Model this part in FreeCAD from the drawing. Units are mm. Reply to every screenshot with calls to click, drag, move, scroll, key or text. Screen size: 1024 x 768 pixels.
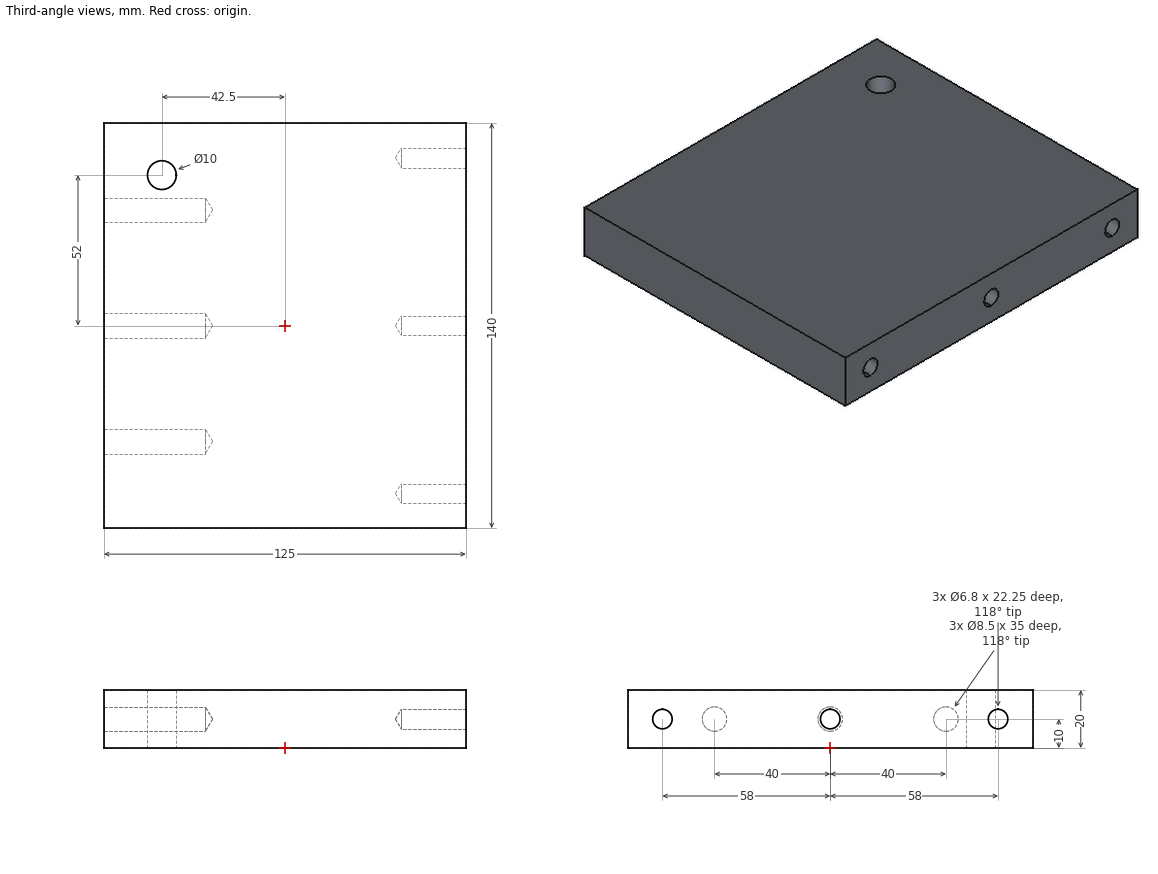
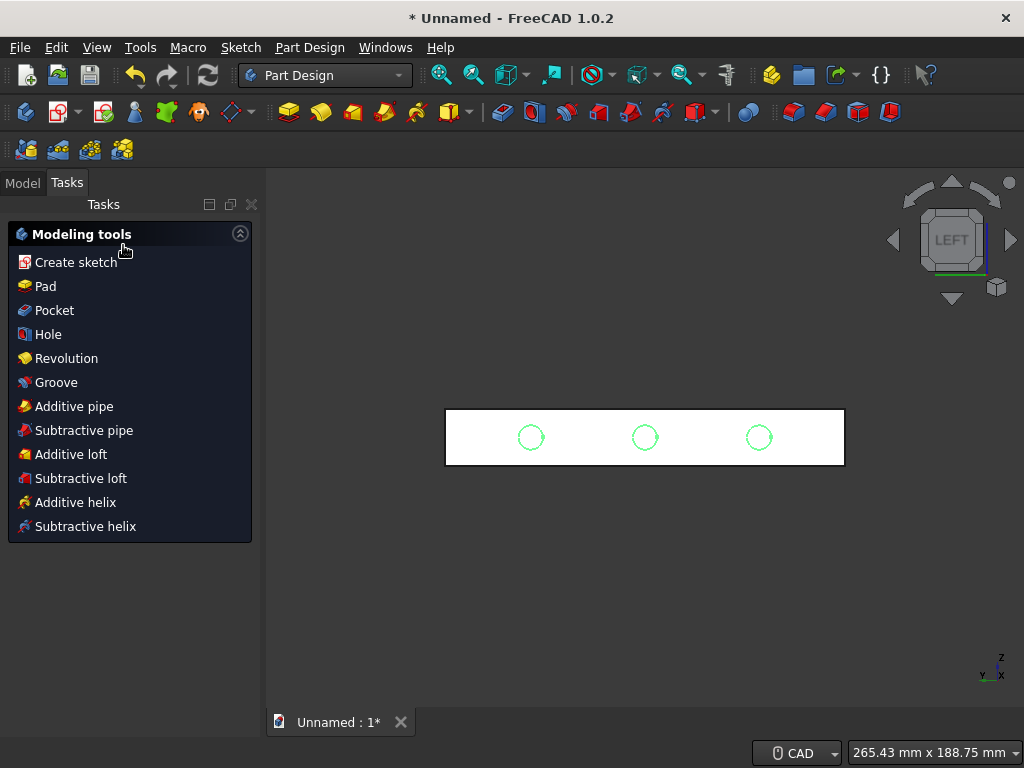
click(536, 112)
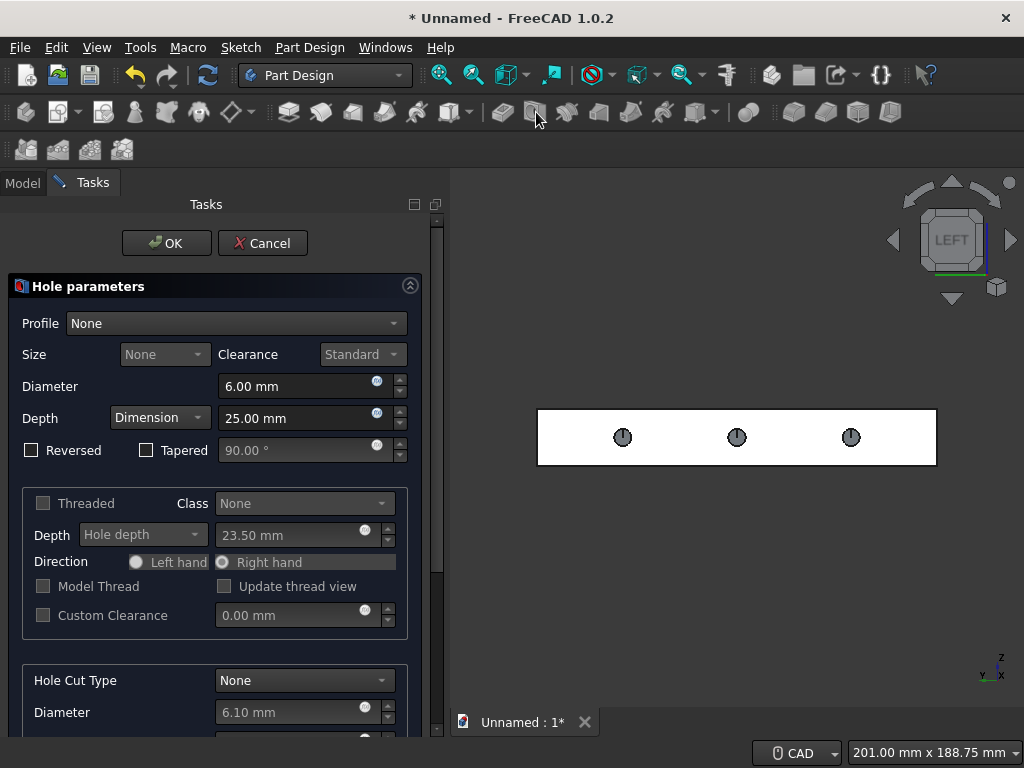
triple_click(305, 386)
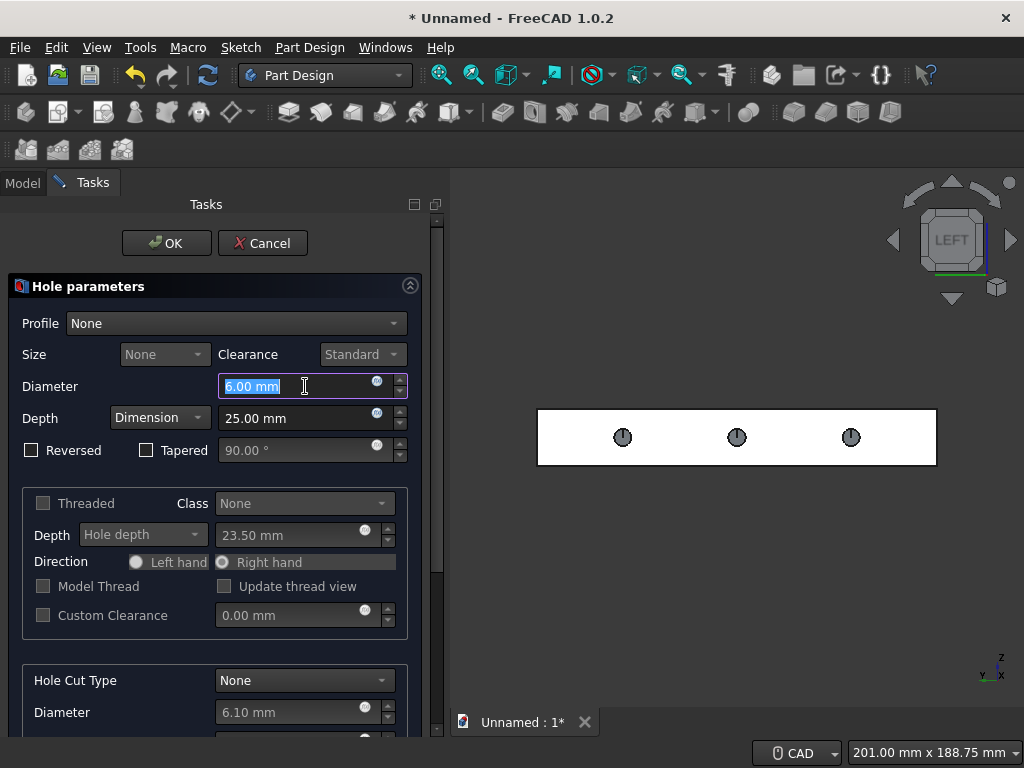
text(8.5)
key(Tab)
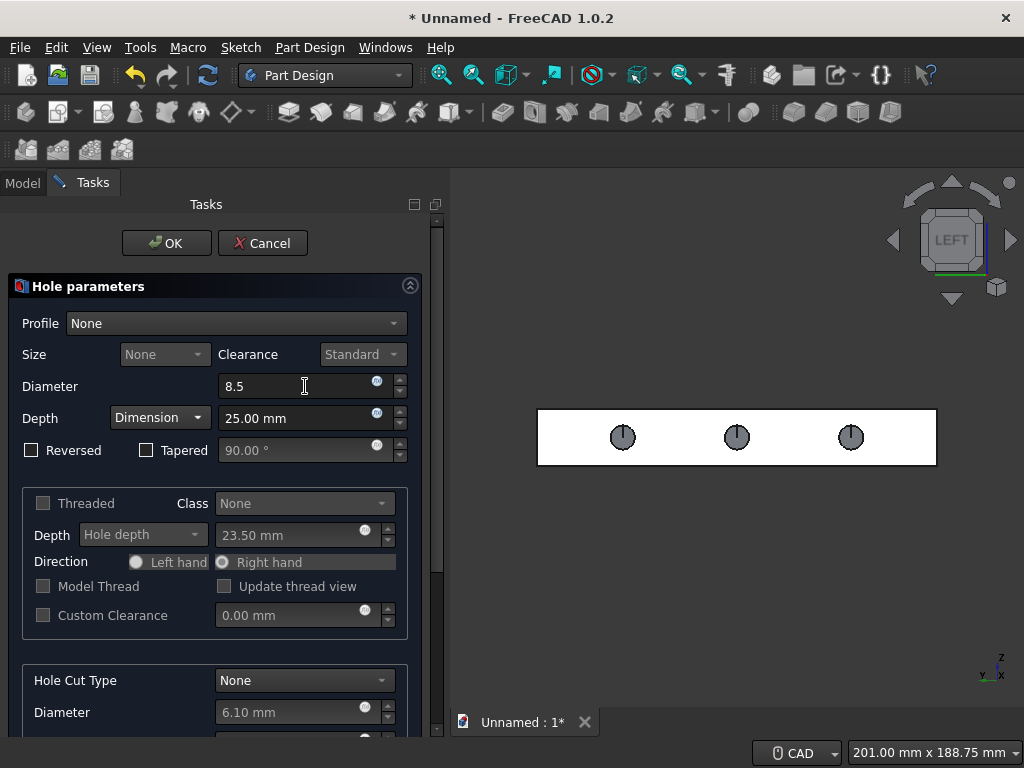
triple_click(305, 418)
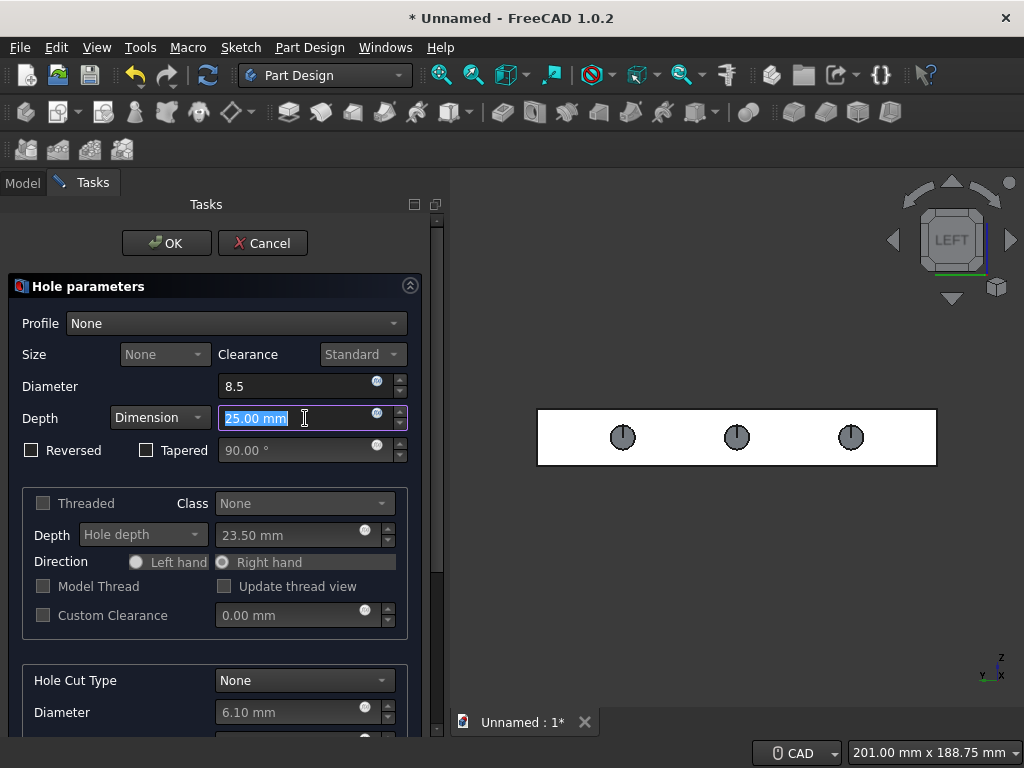
text(35)
key(Tab)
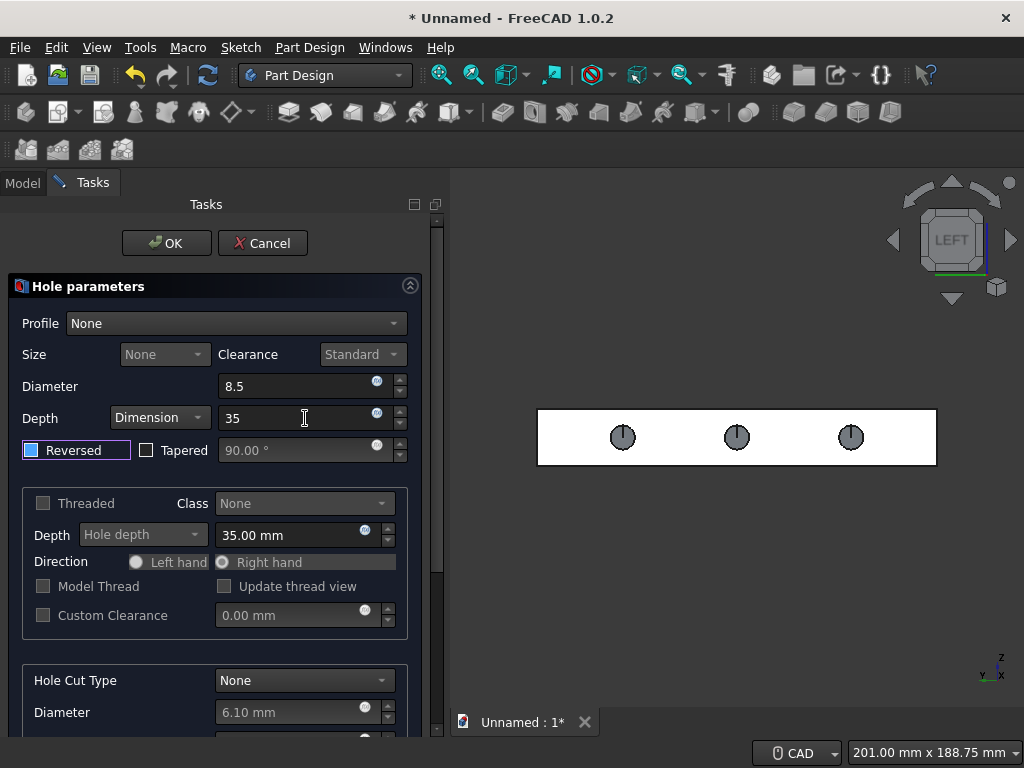
click(167, 243)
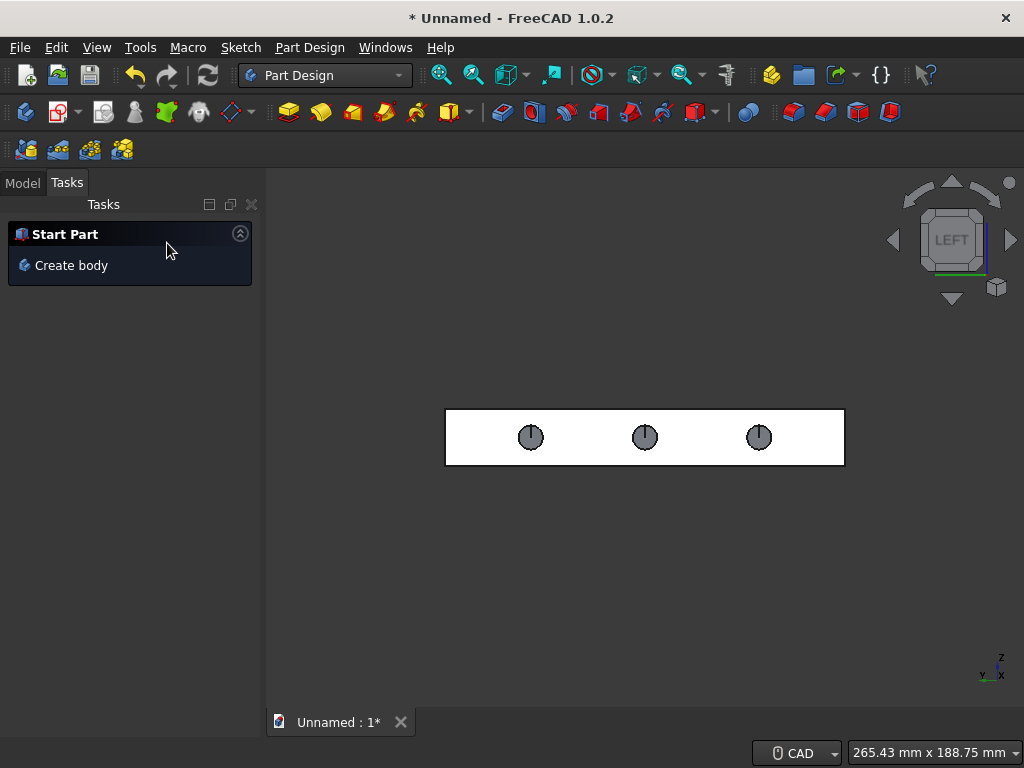
key(0)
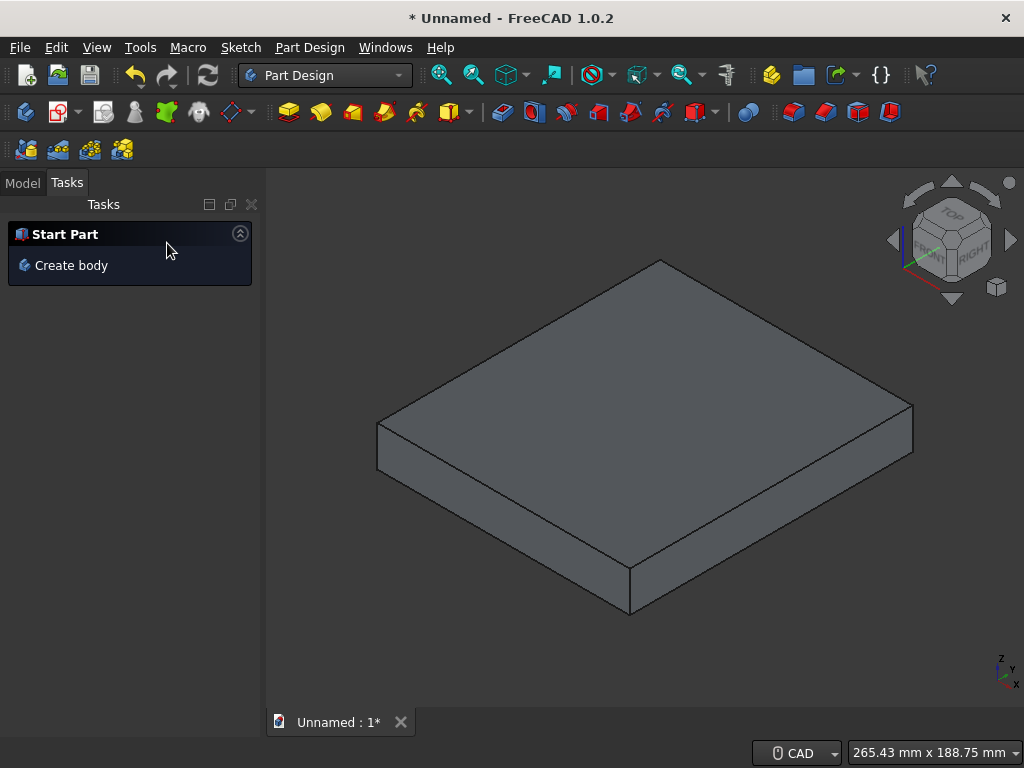
click(892, 439)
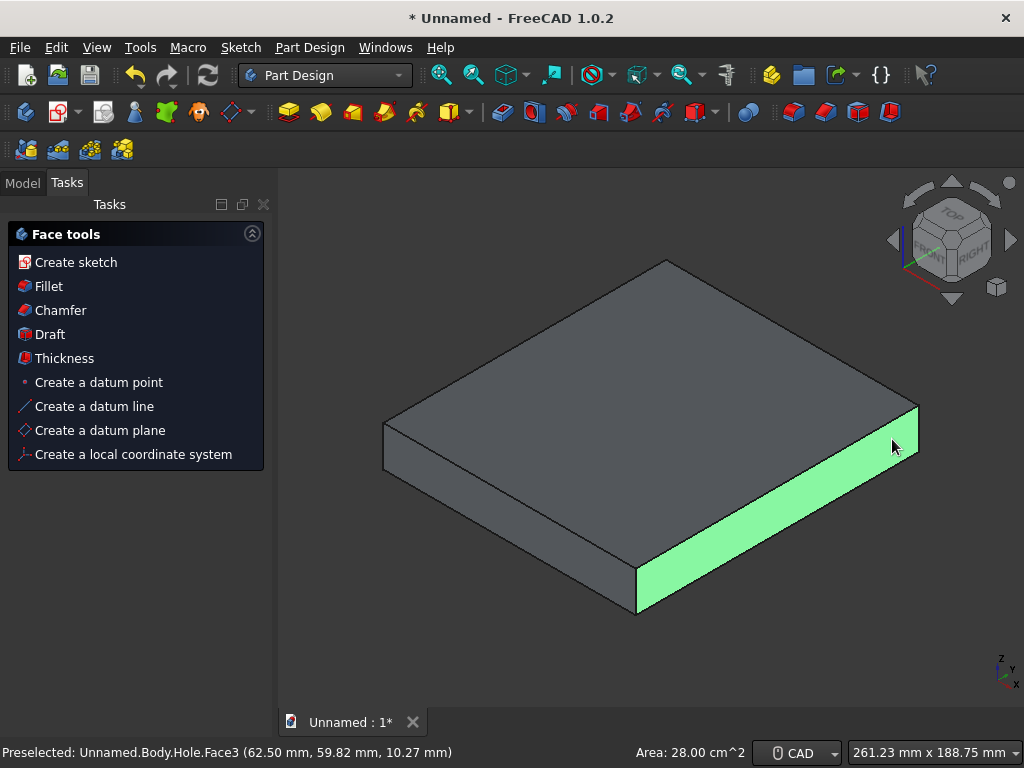
click(58, 112)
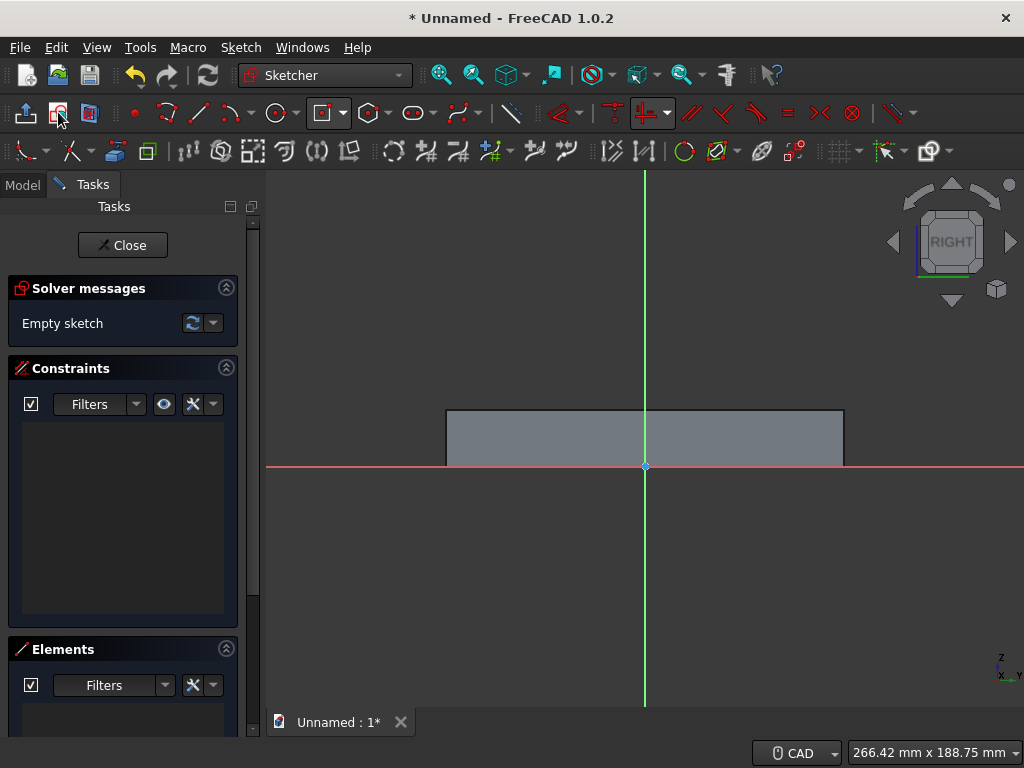
click(276, 114)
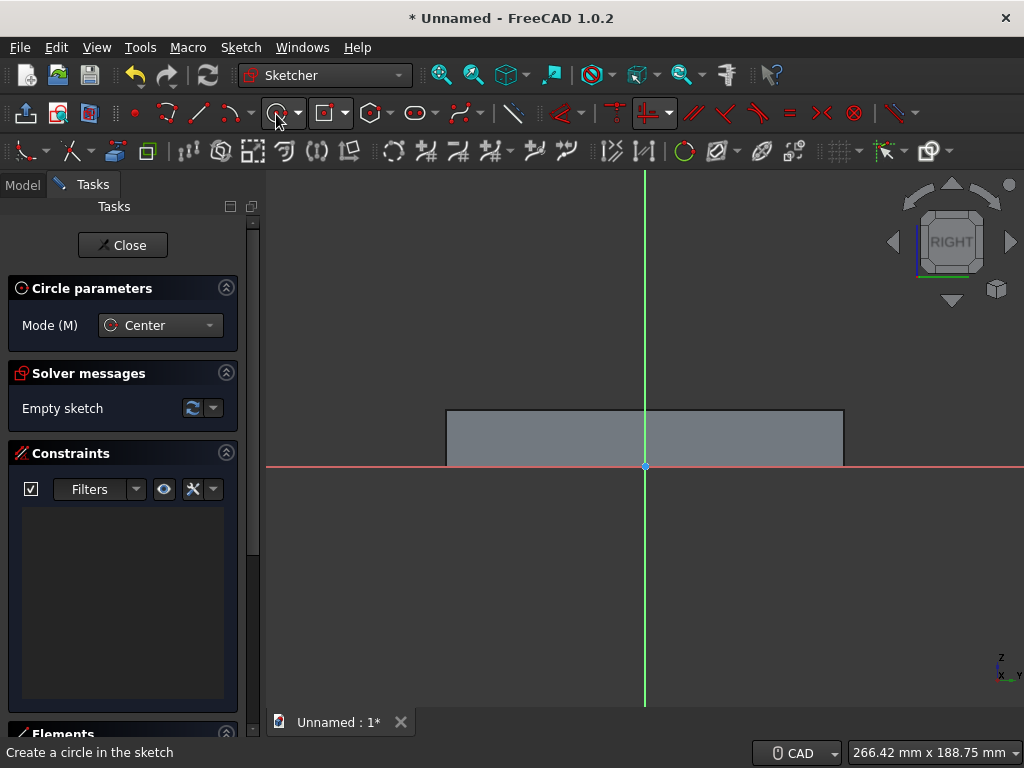
scroll(810, 439, up, 5)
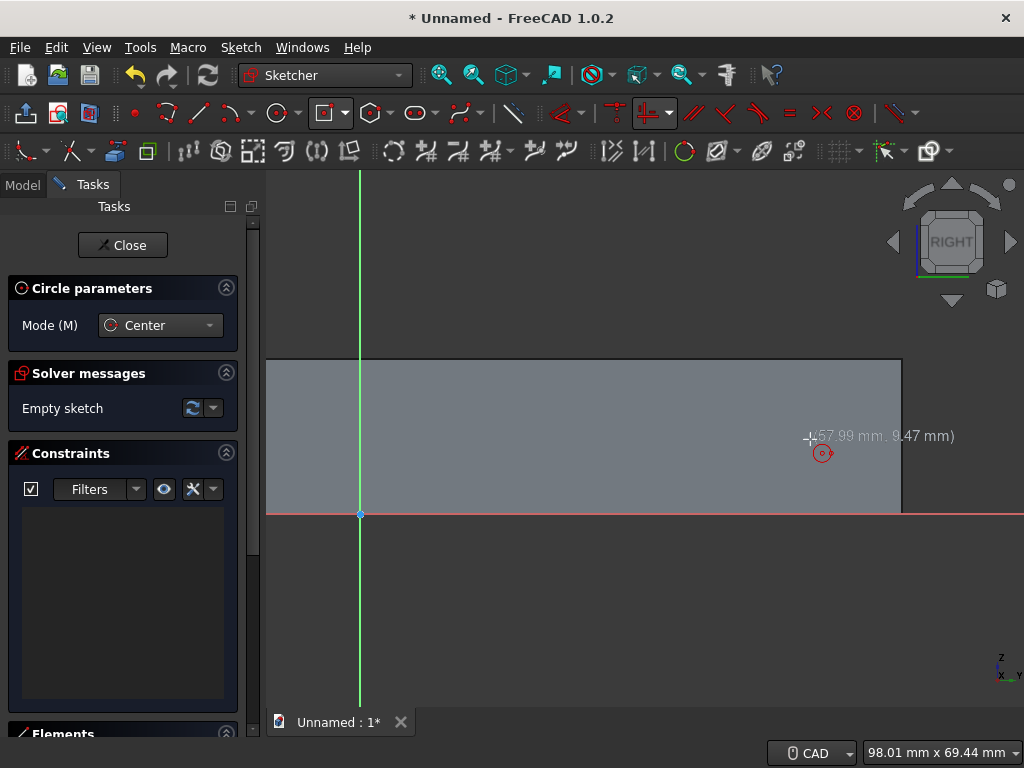
click(809, 437)
click(827, 418)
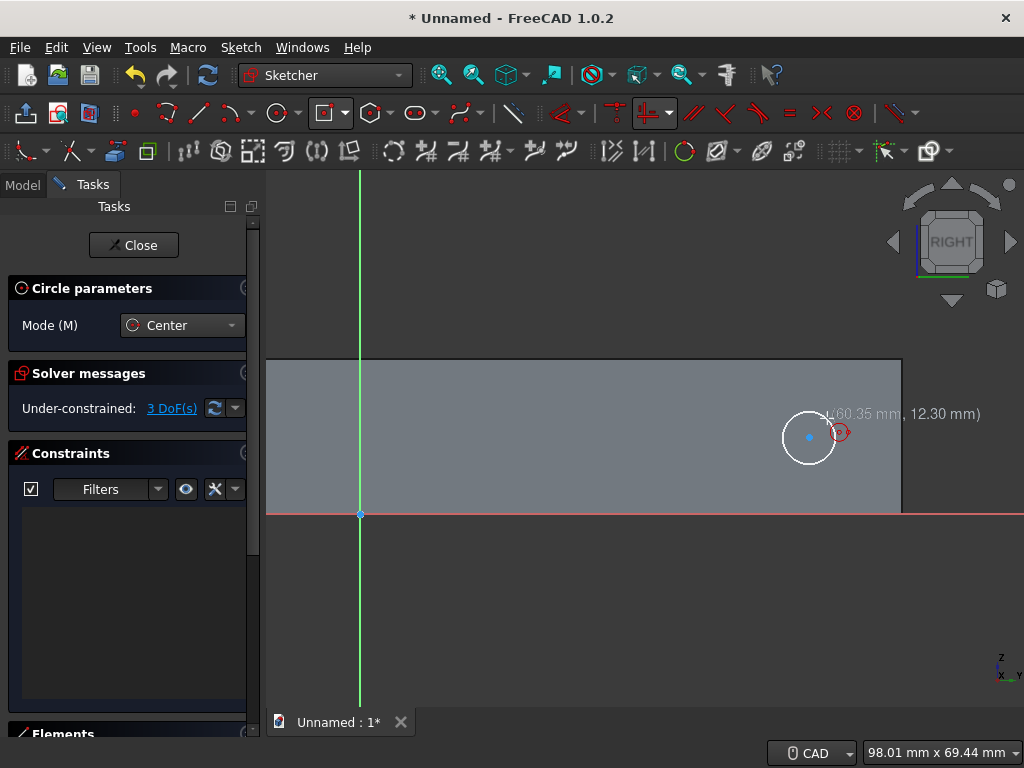
click(360, 437)
click(379, 418)